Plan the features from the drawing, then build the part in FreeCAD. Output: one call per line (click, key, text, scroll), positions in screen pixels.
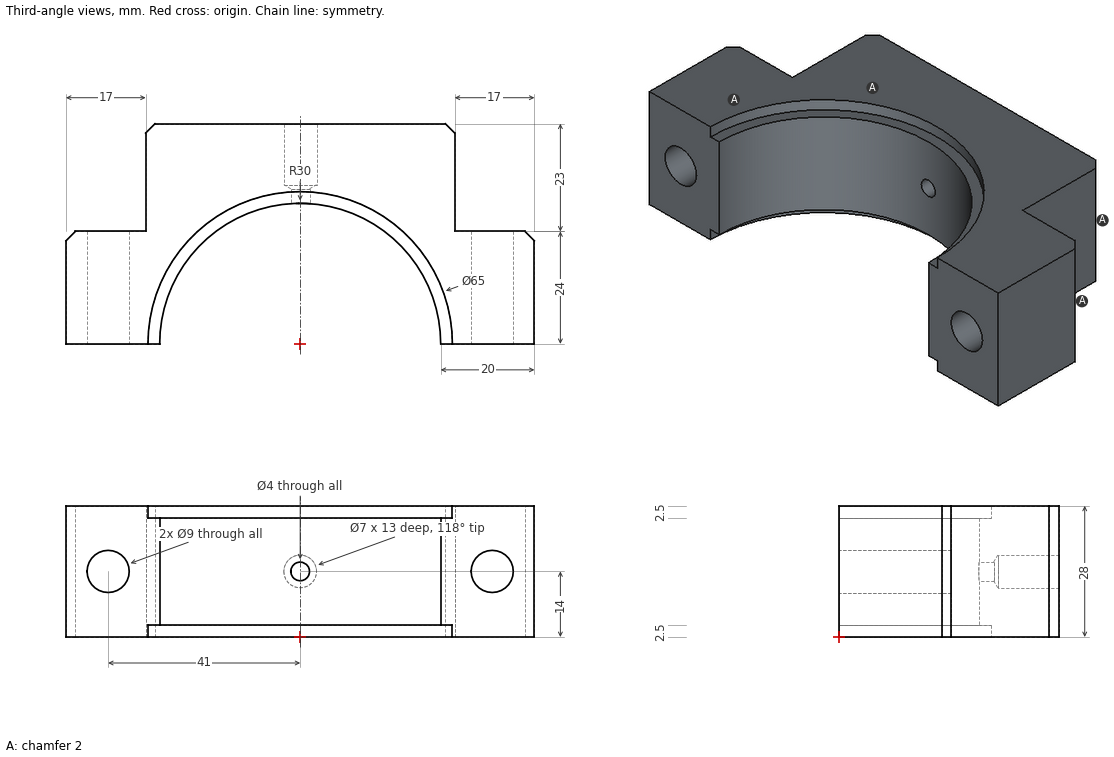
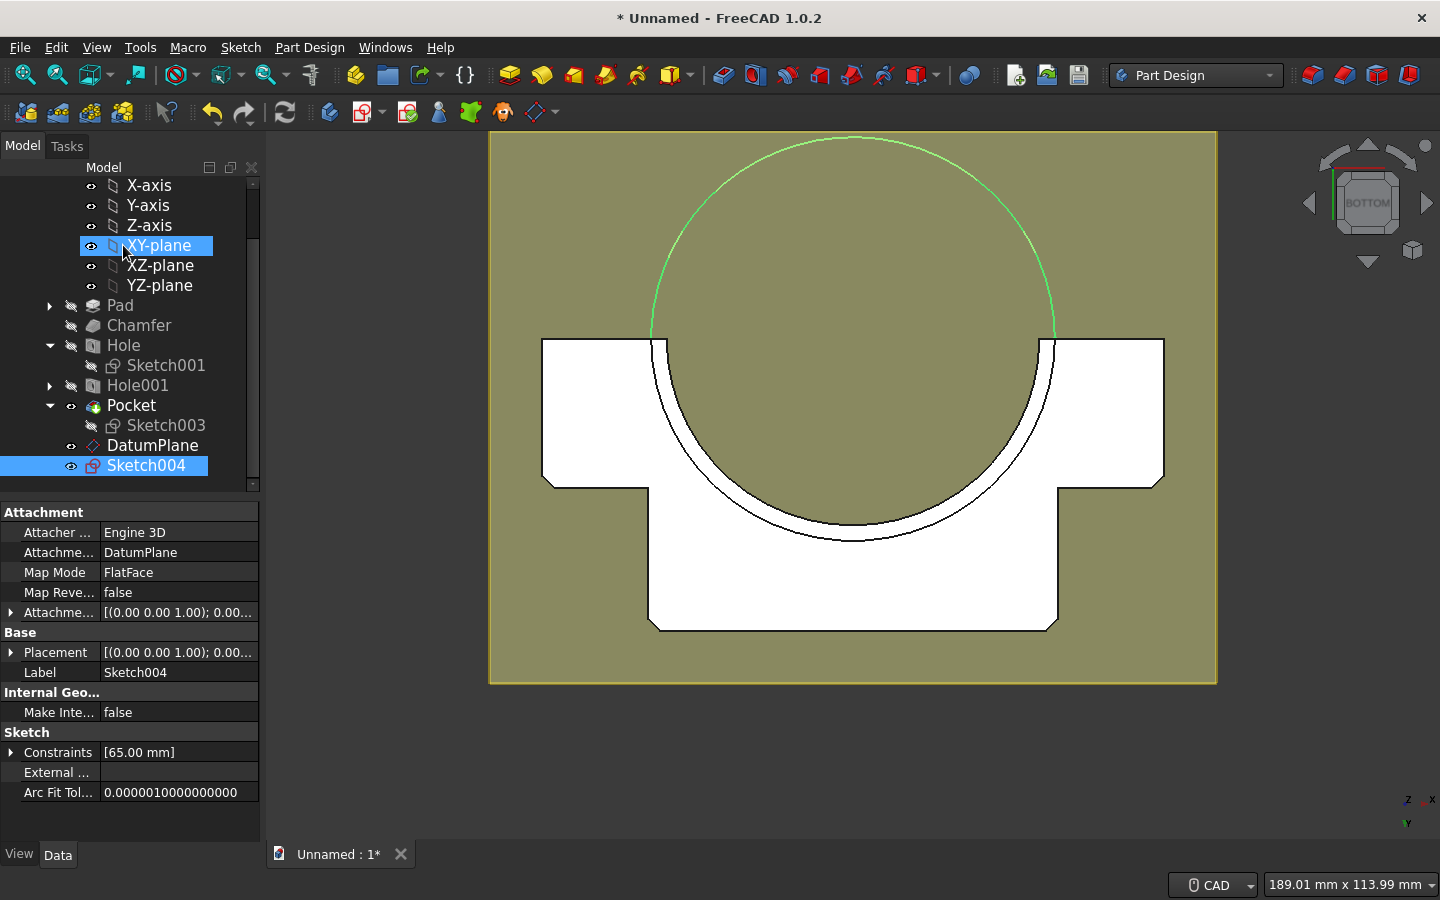
click(724, 76)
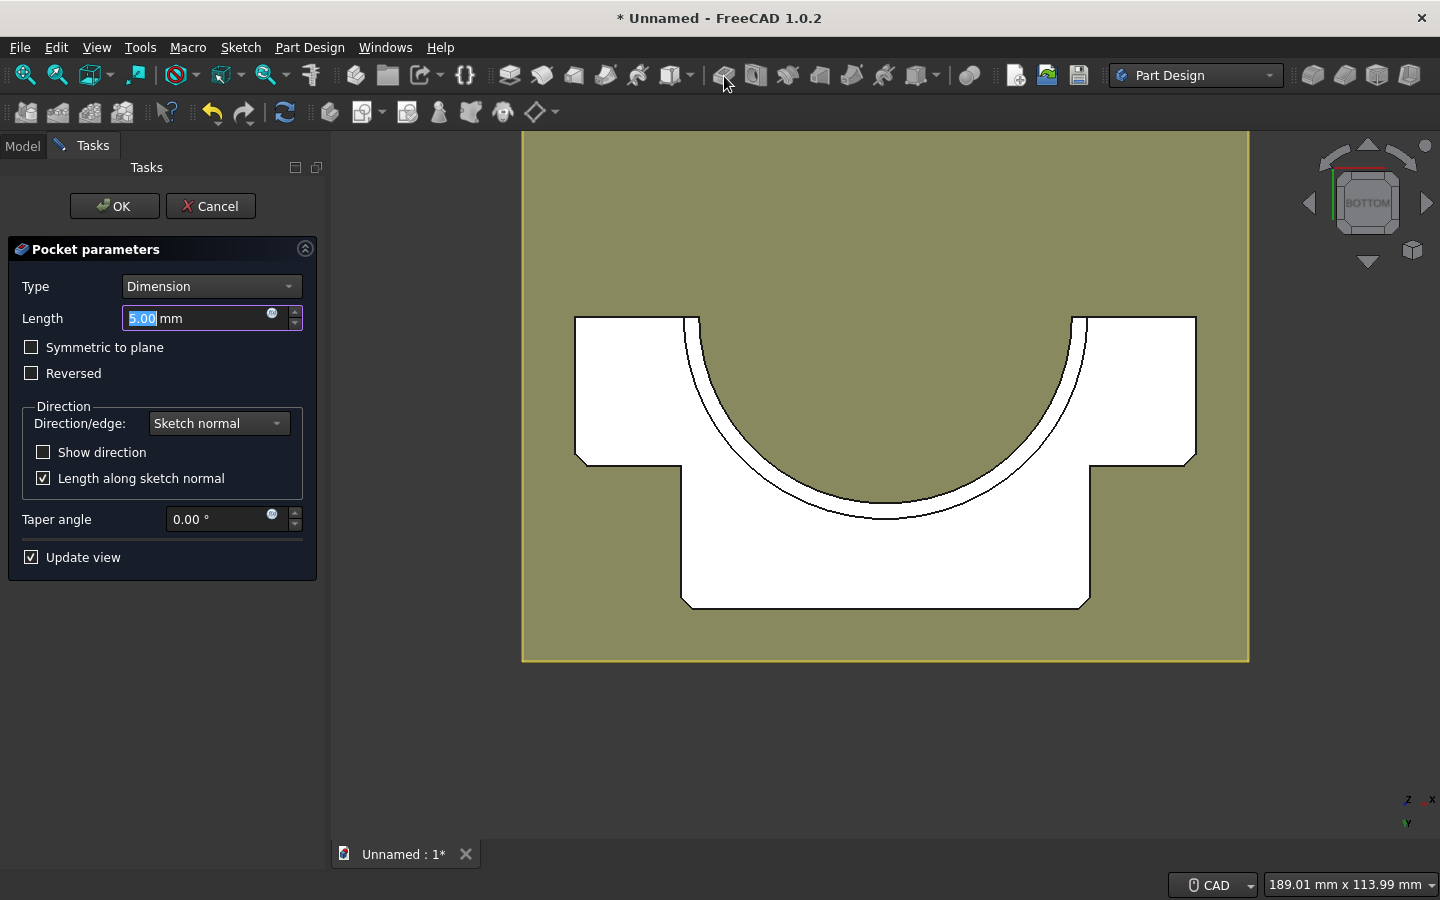
text(2.5)
key(Tab)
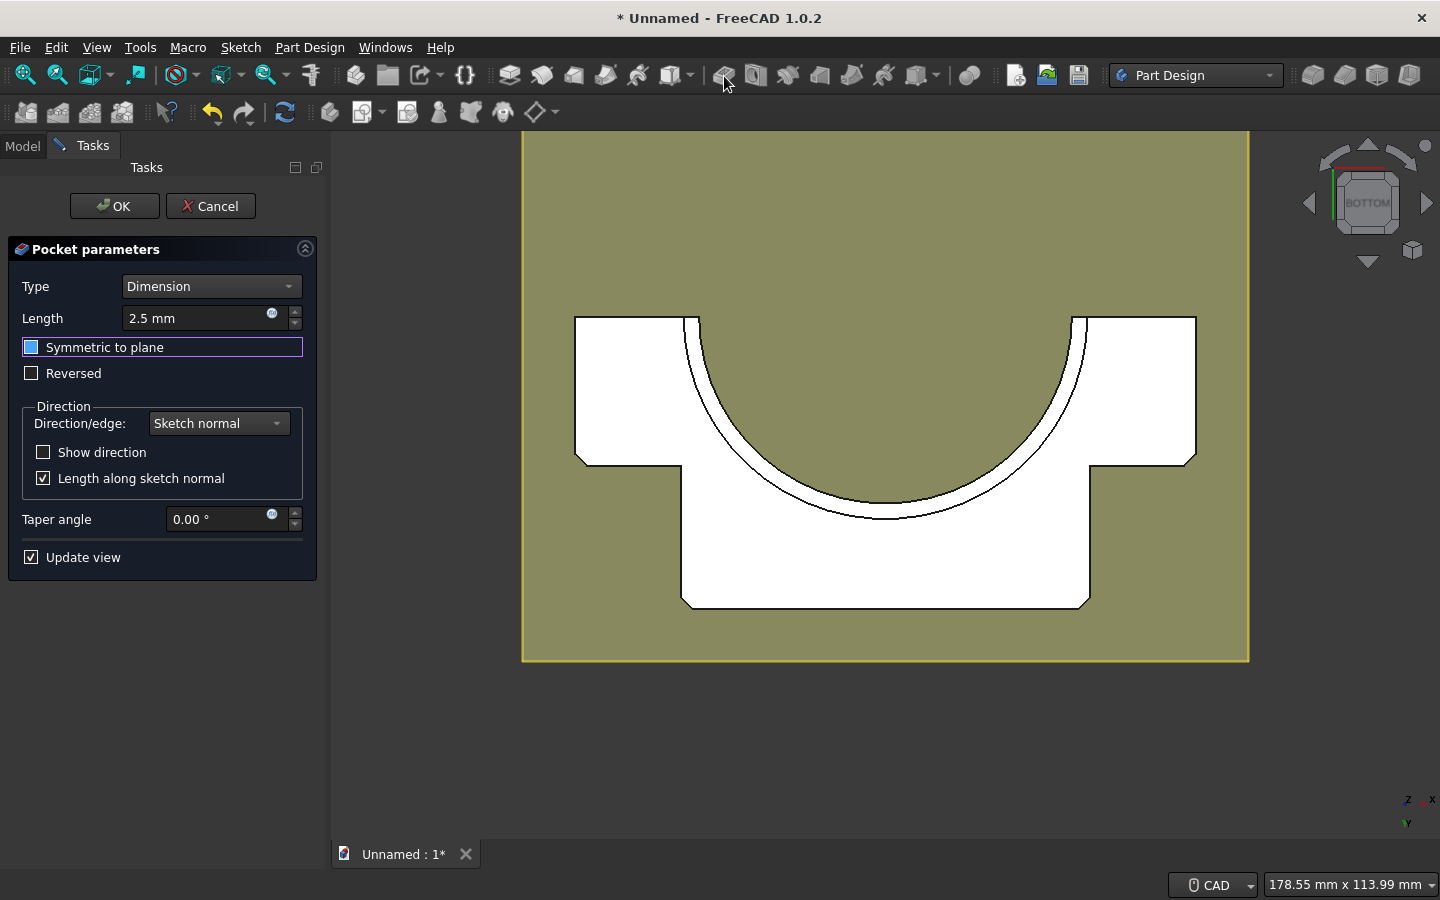
click(30, 373)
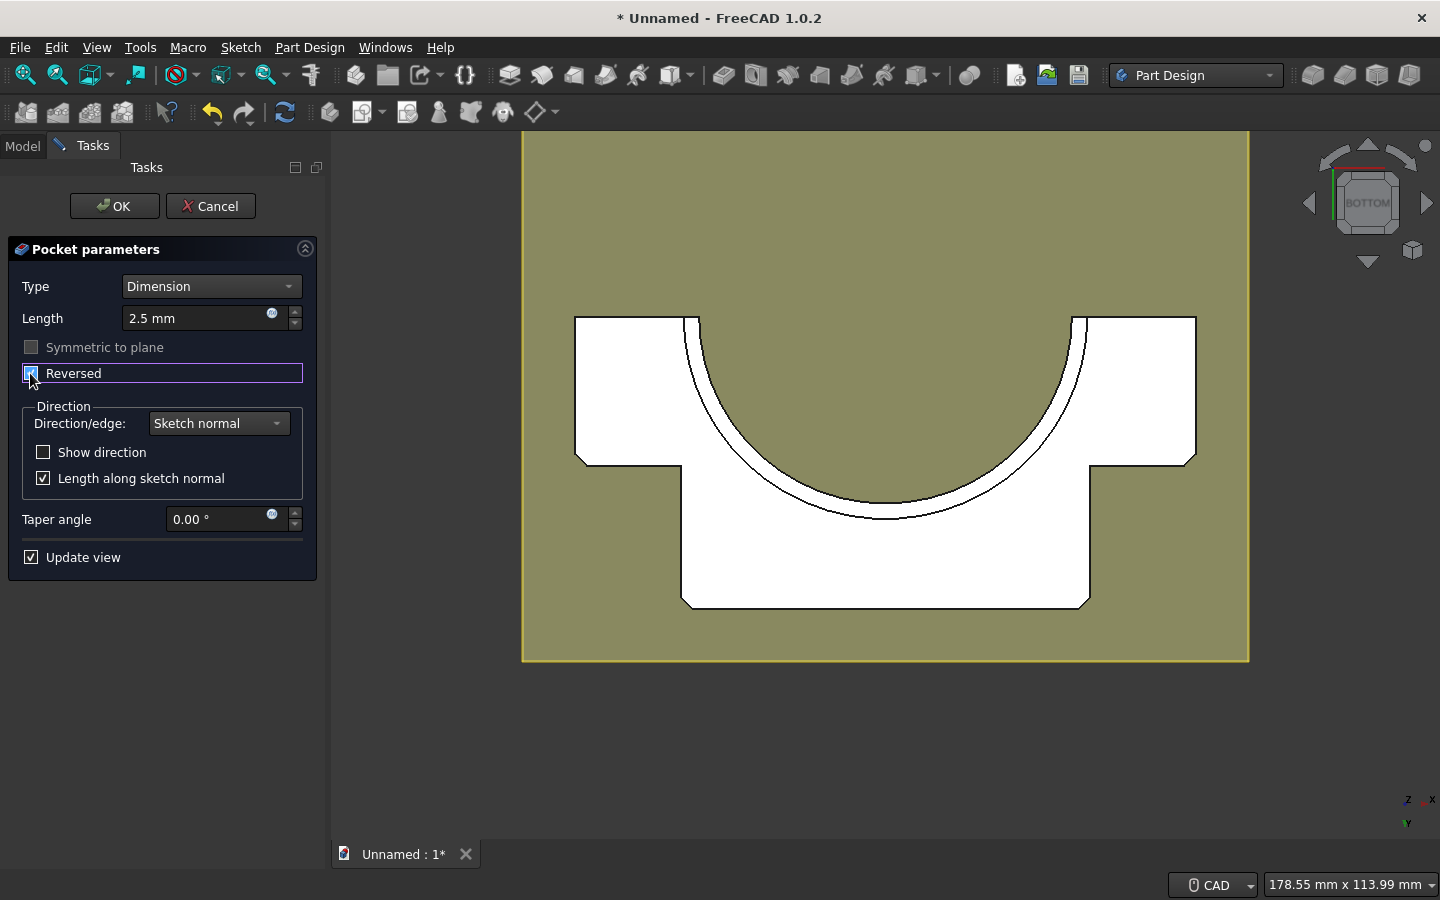
click(115, 206)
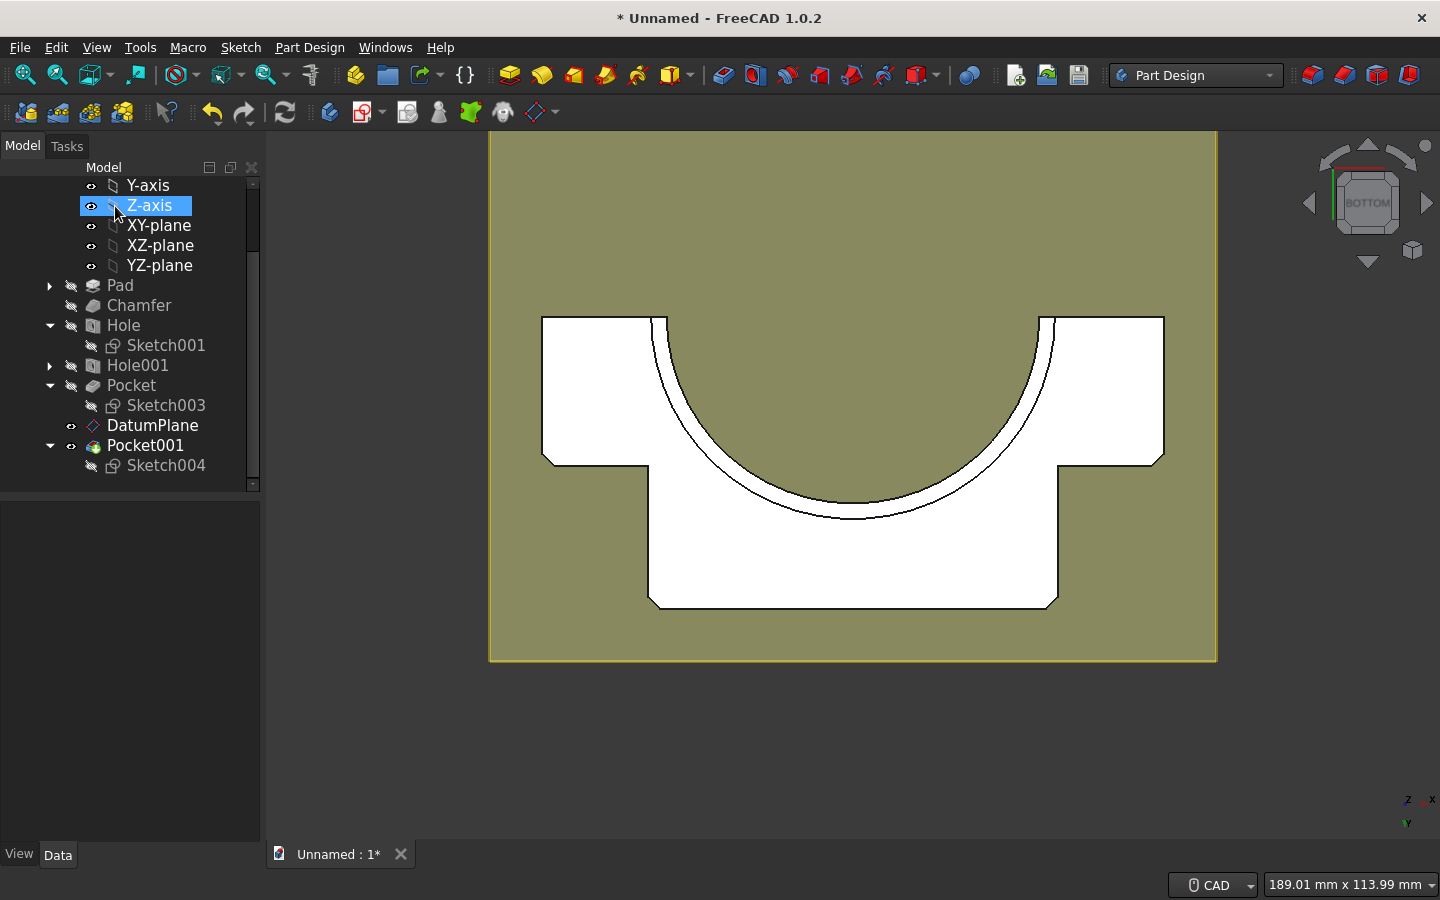
click(116, 426)
key(space)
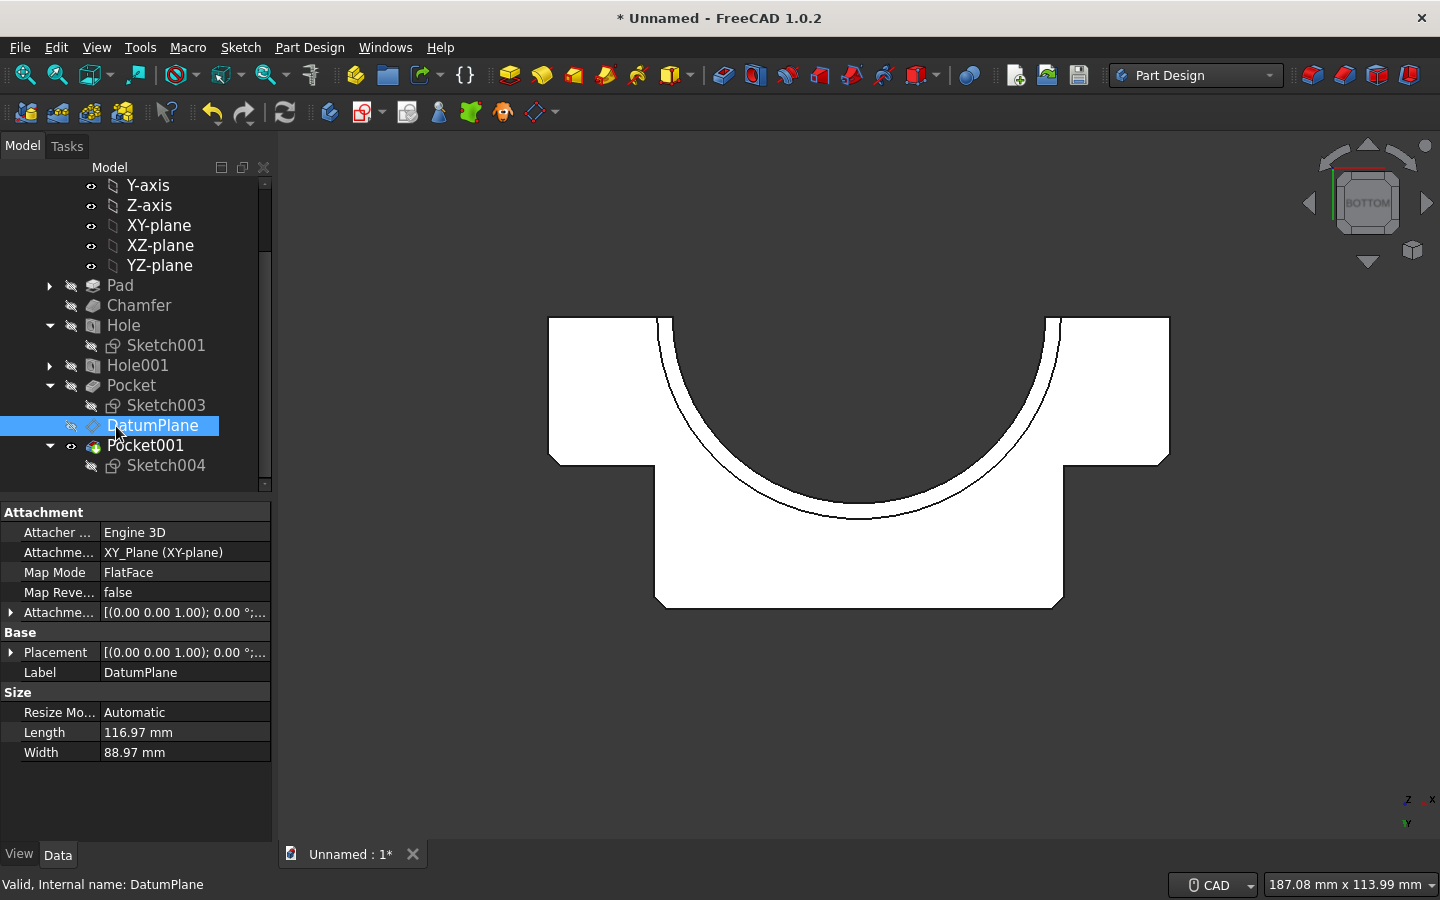
key(4)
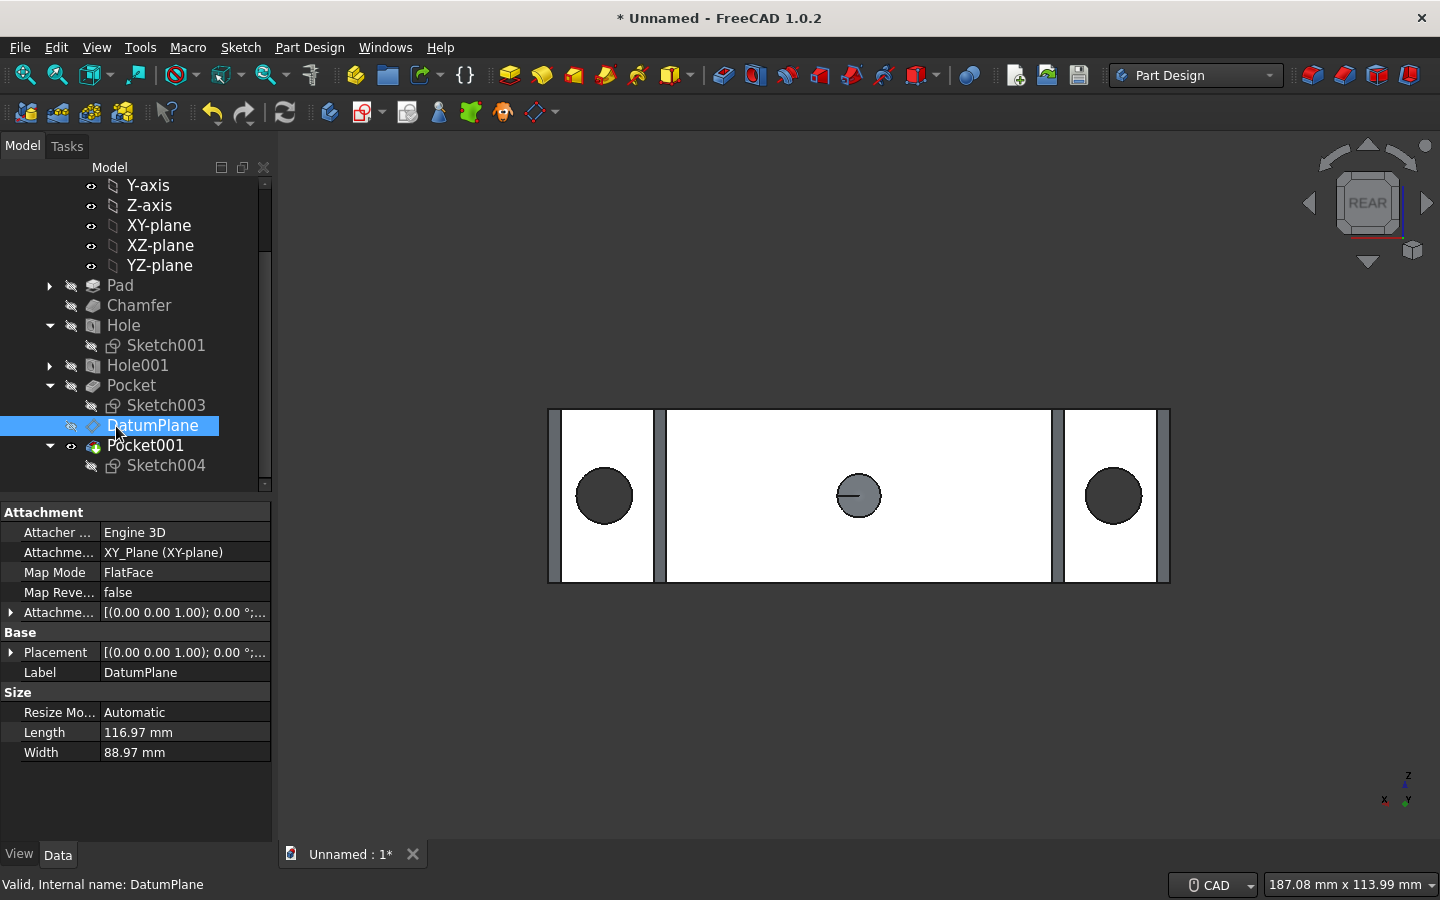
click(749, 495)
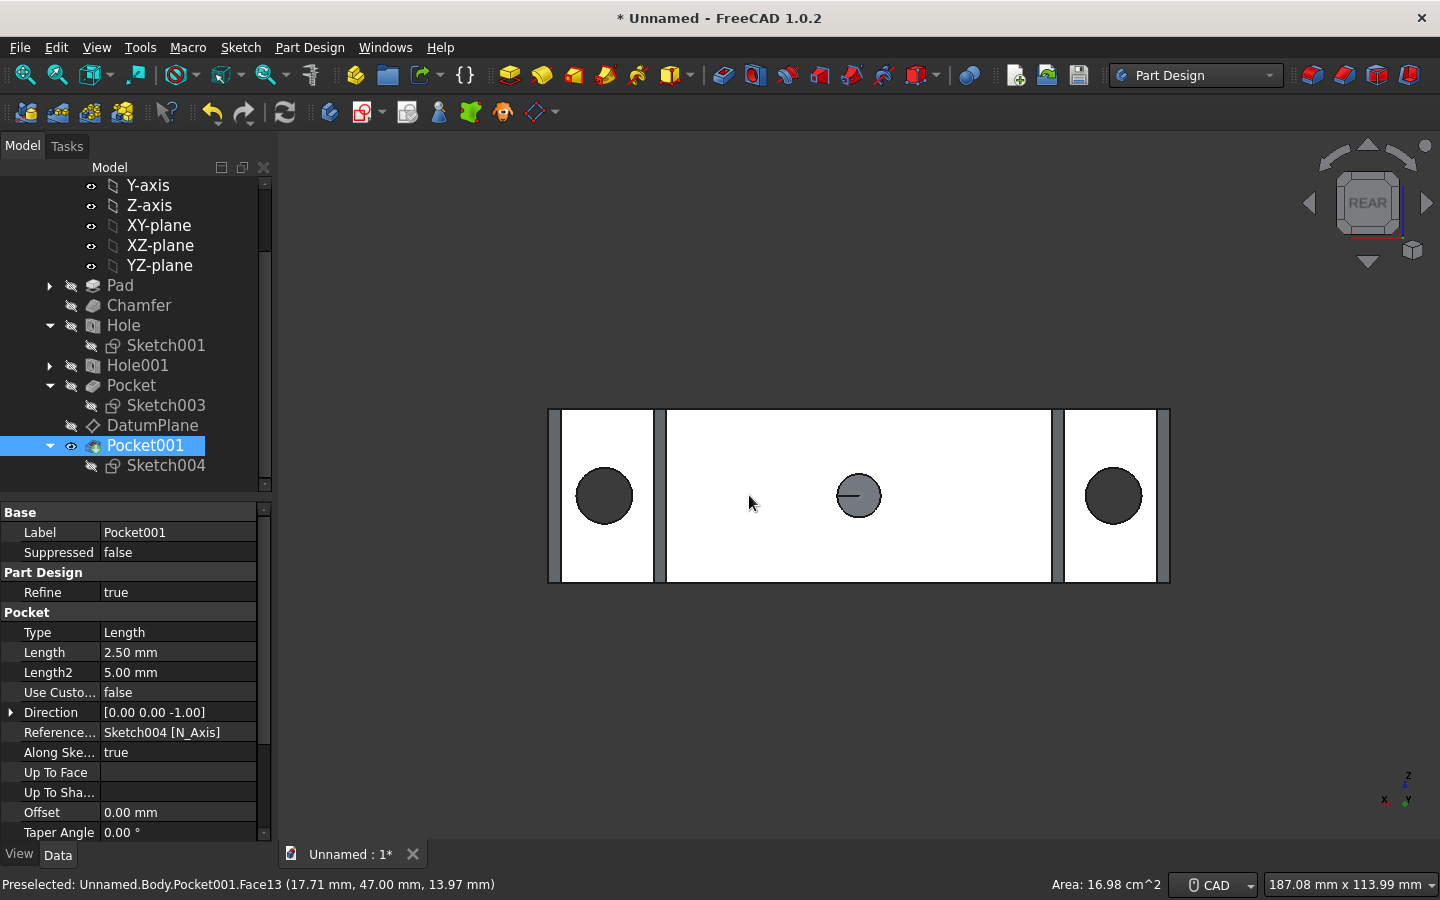
click(362, 112)